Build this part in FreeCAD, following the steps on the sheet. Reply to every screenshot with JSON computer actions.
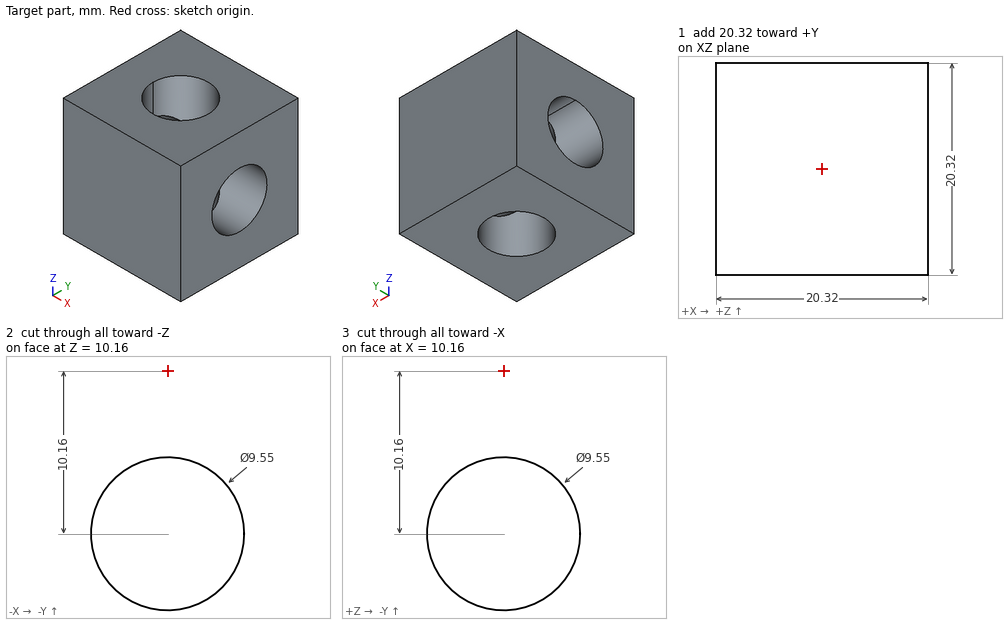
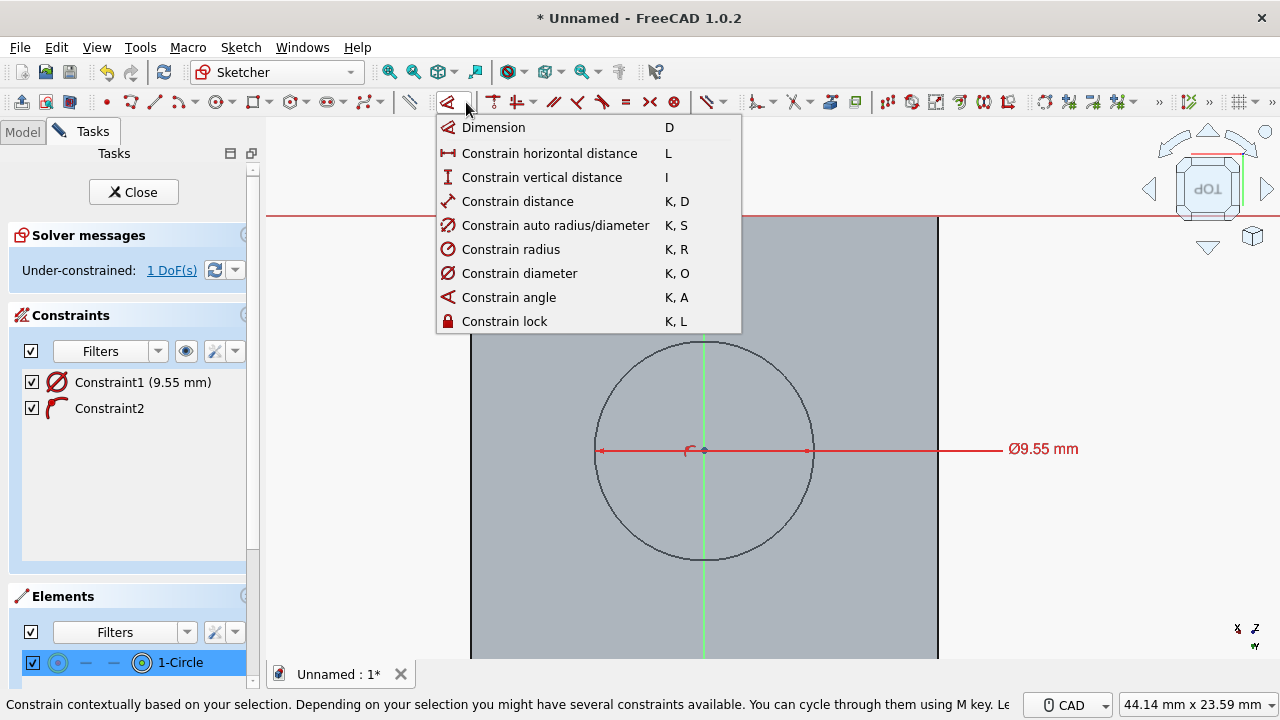
{"action": "left_click", "coordinate": [589, 177]}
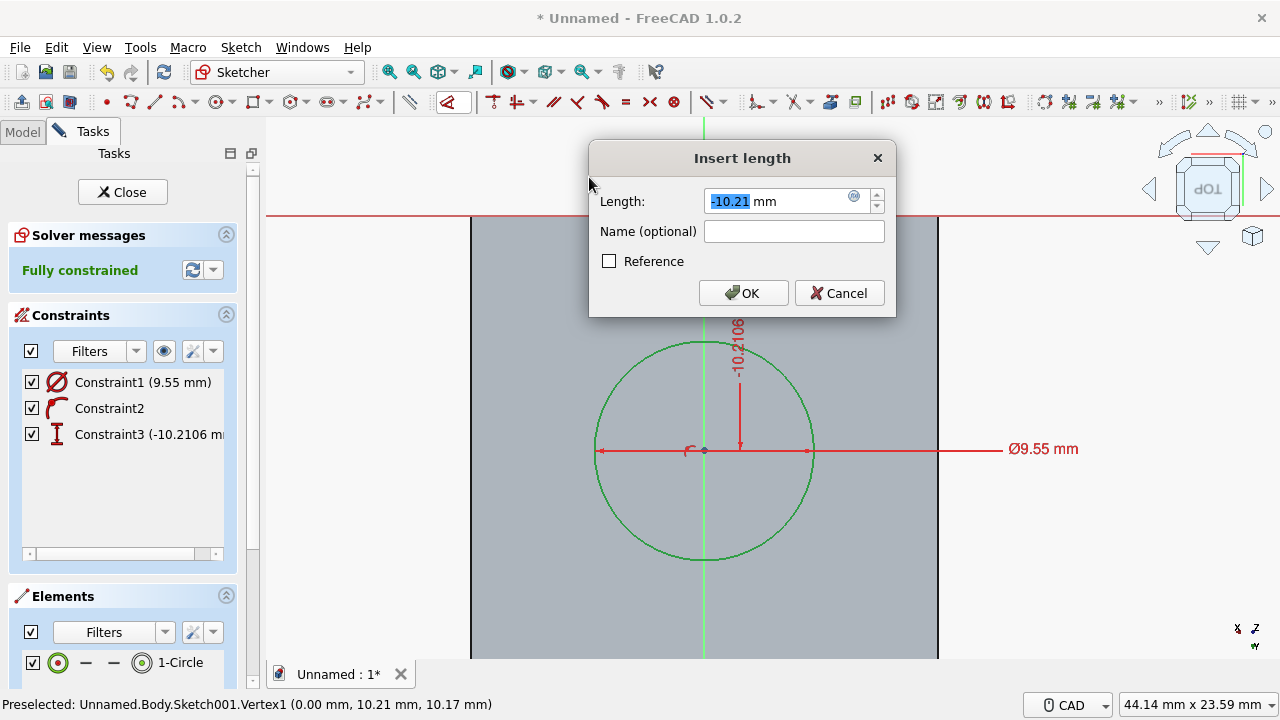
{"action": "type", "text": "-10.16"}
{"action": "key", "text": "Return"}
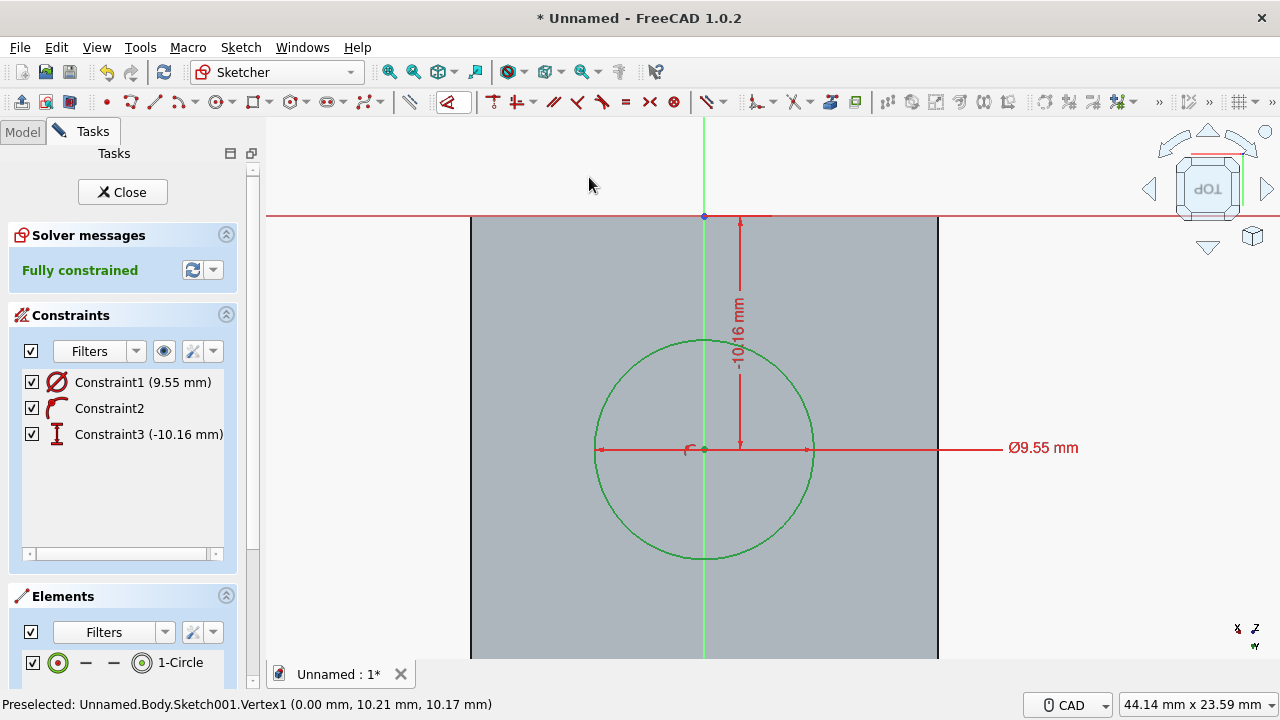
{"action": "left_click", "coordinate": [123, 192]}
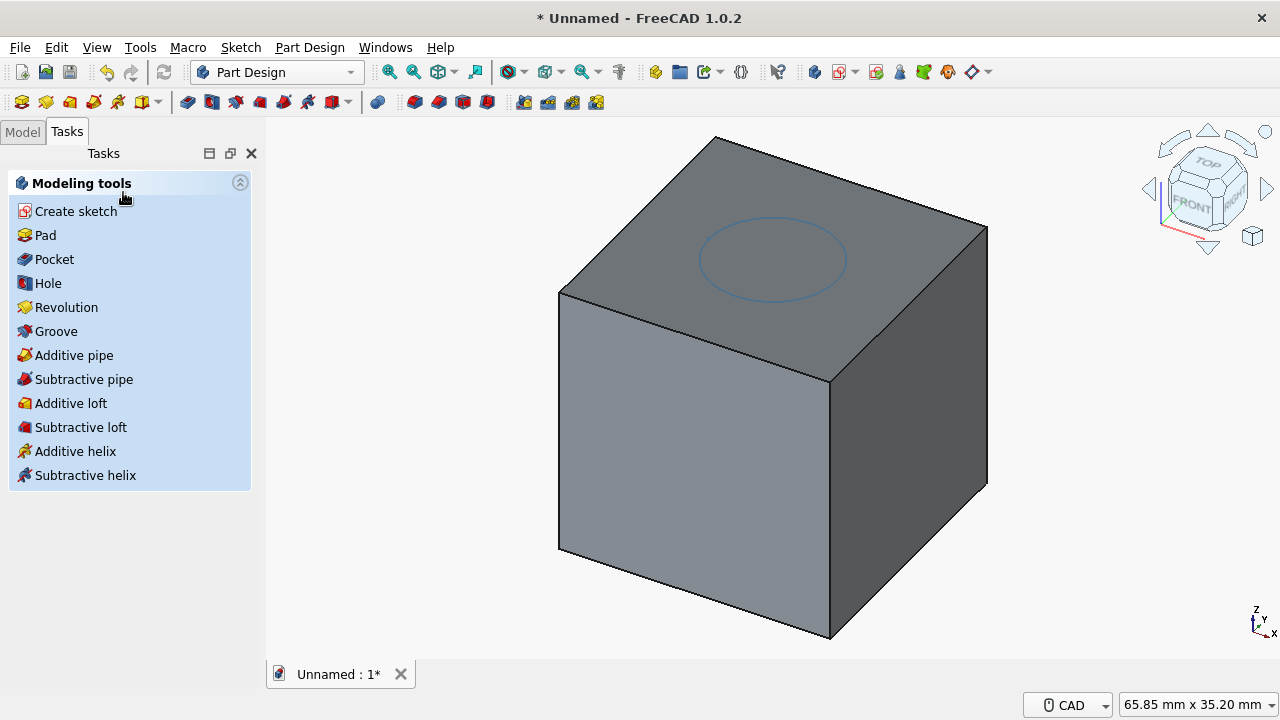
{"action": "left_click", "coordinate": [188, 102]}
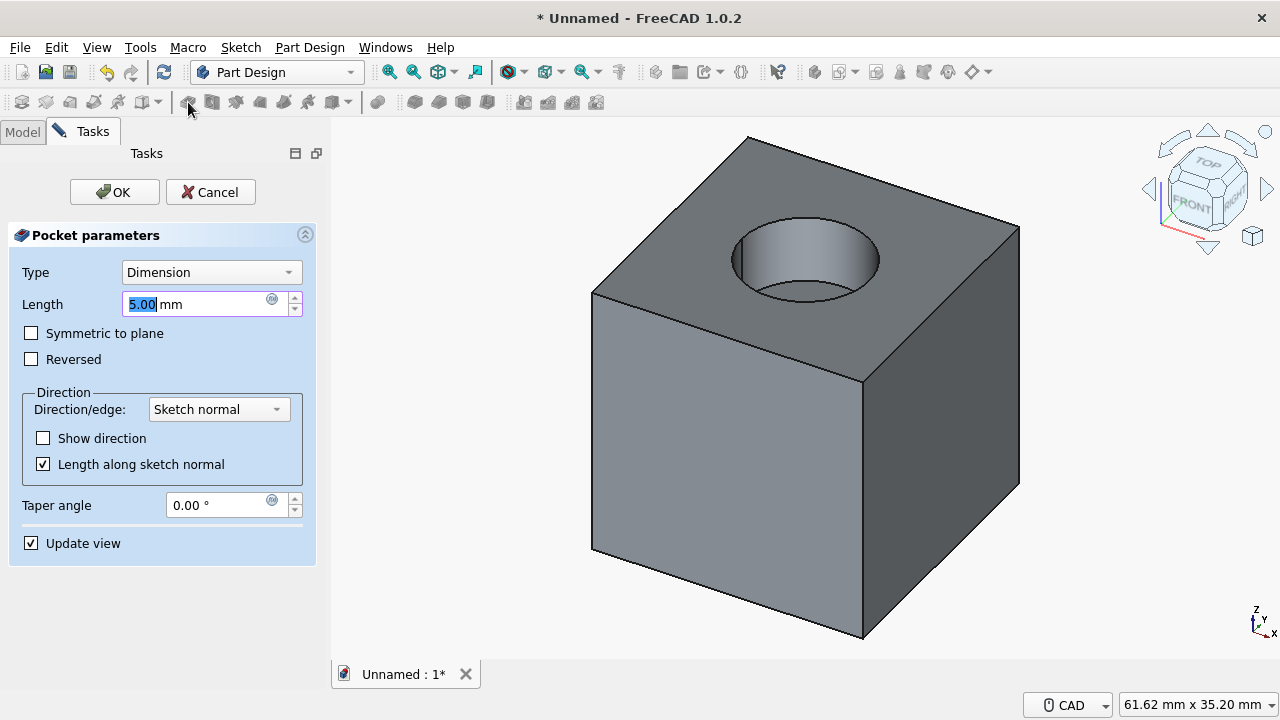
{"action": "left_click", "coordinate": [212, 272]}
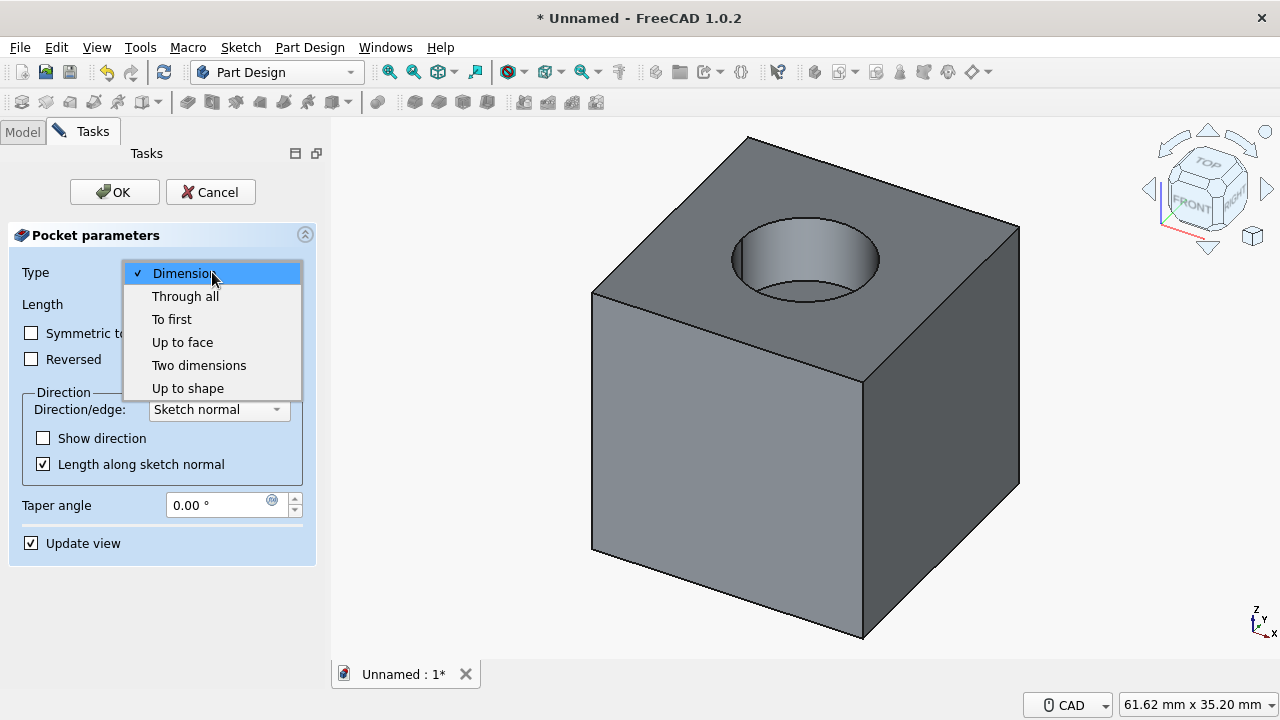
{"action": "left_click", "coordinate": [212, 296]}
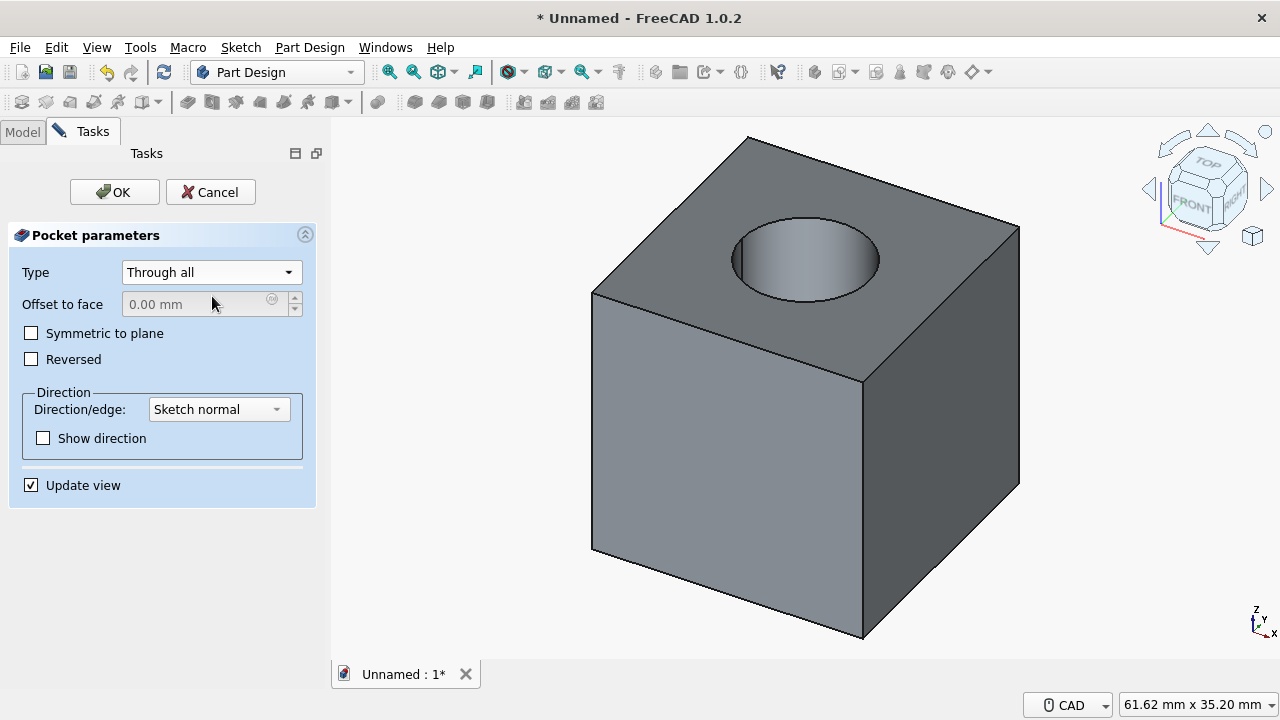
{"action": "left_click", "coordinate": [115, 192]}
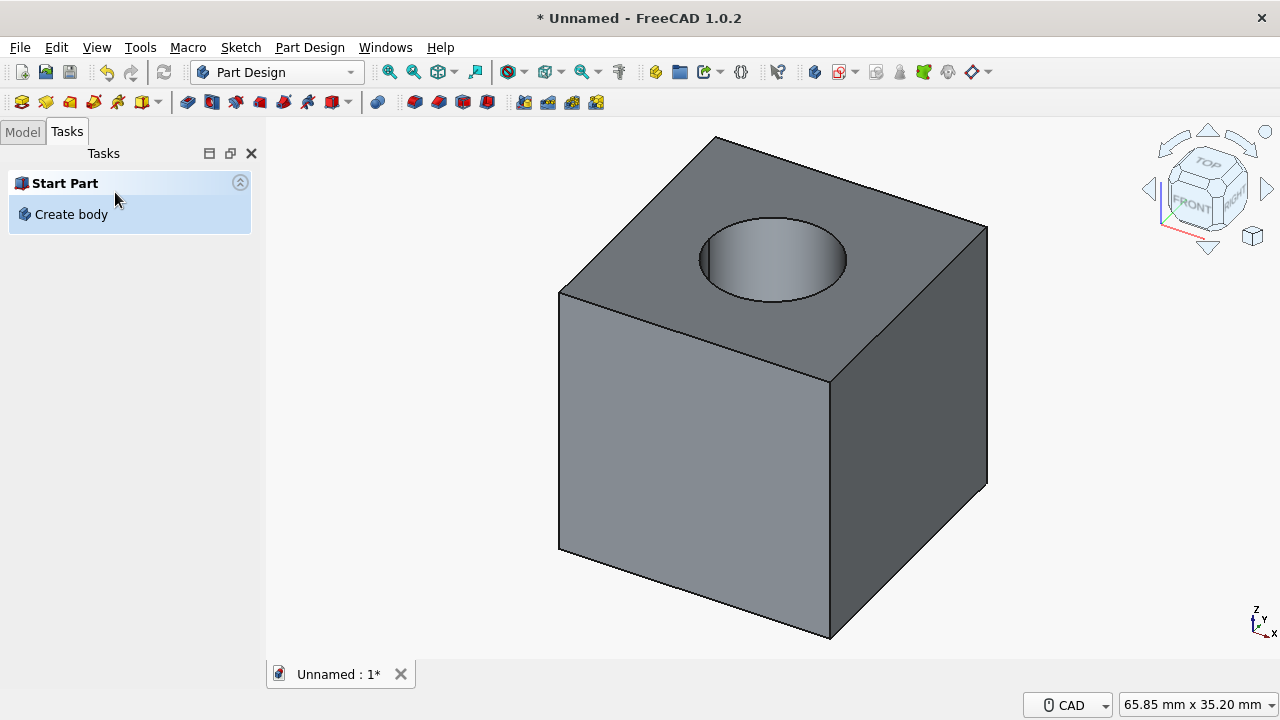
{"action": "left_click", "coordinate": [909, 432]}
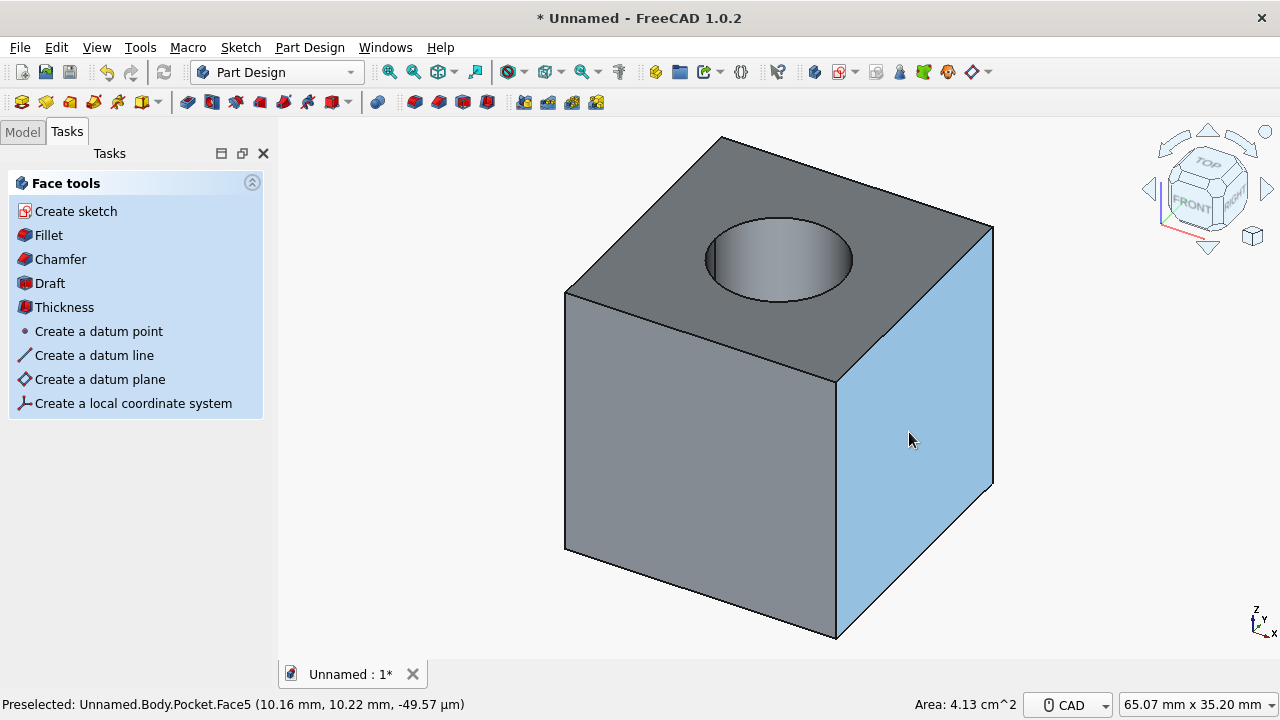
{"action": "left_click", "coordinate": [840, 72]}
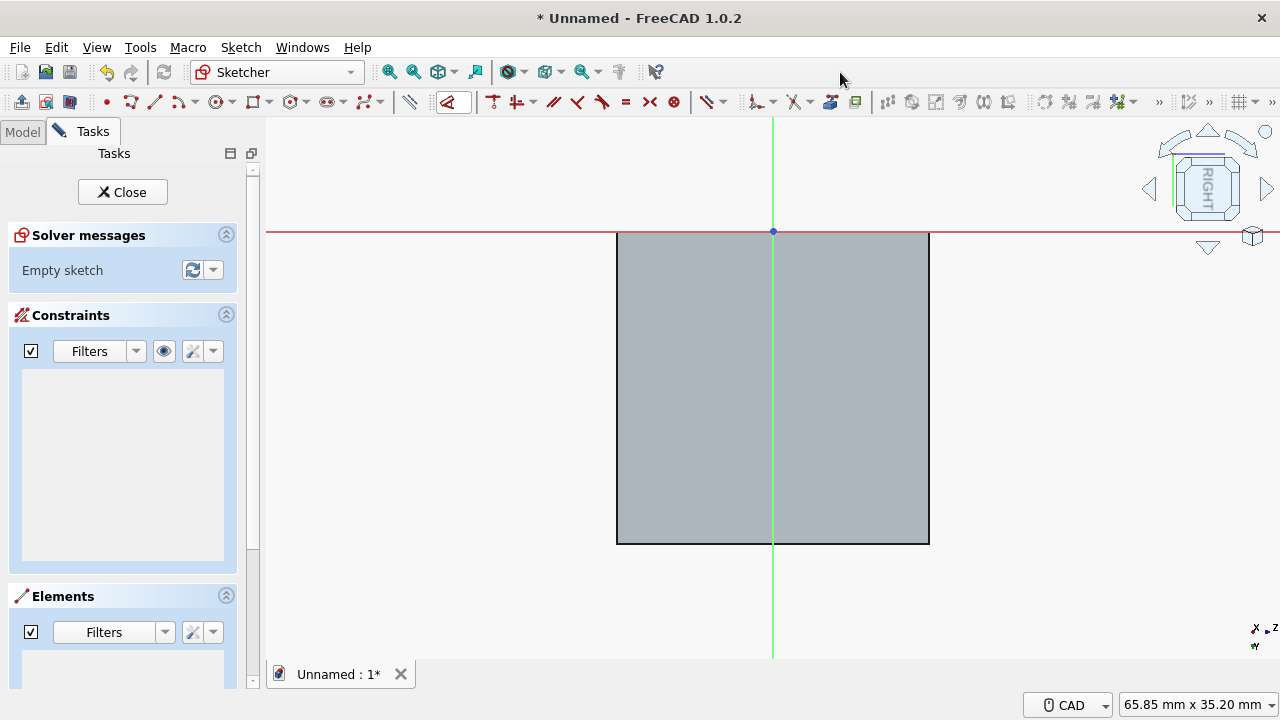
{"action": "scroll", "coordinate": [912, 262], "scroll_direction": "up", "scroll_amount": 2}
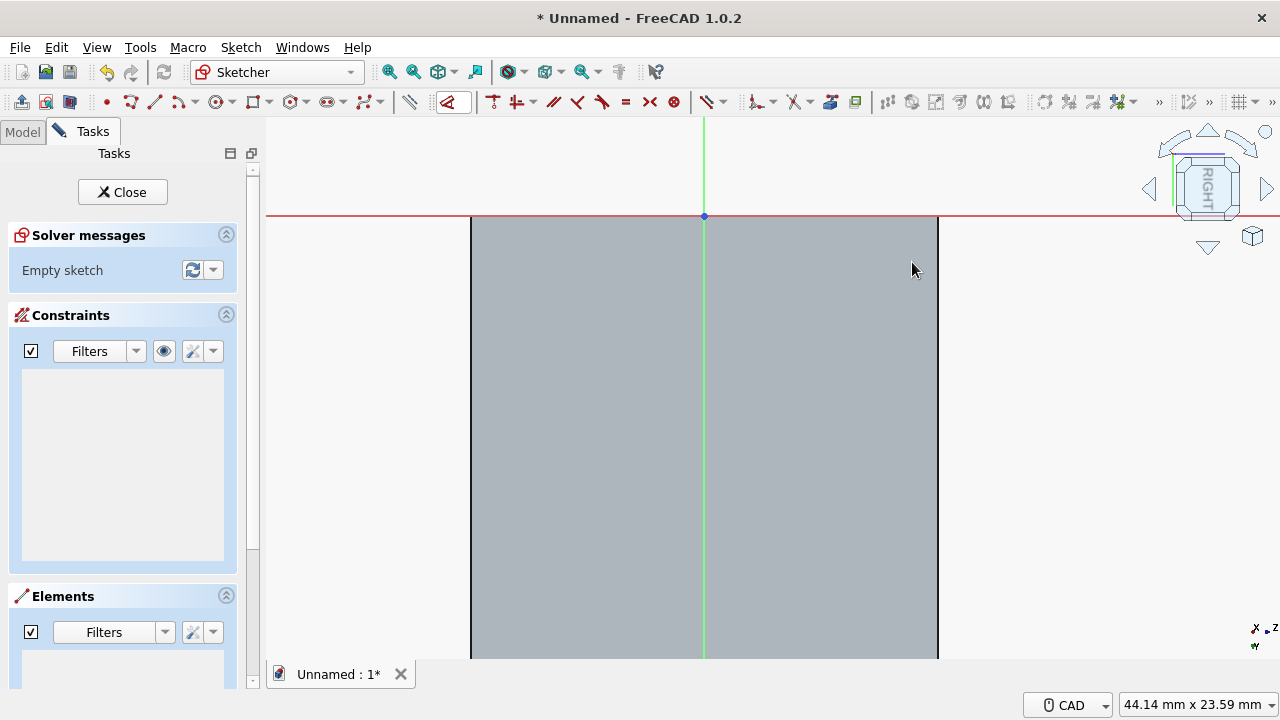
{"action": "left_click", "coordinate": [216, 102]}